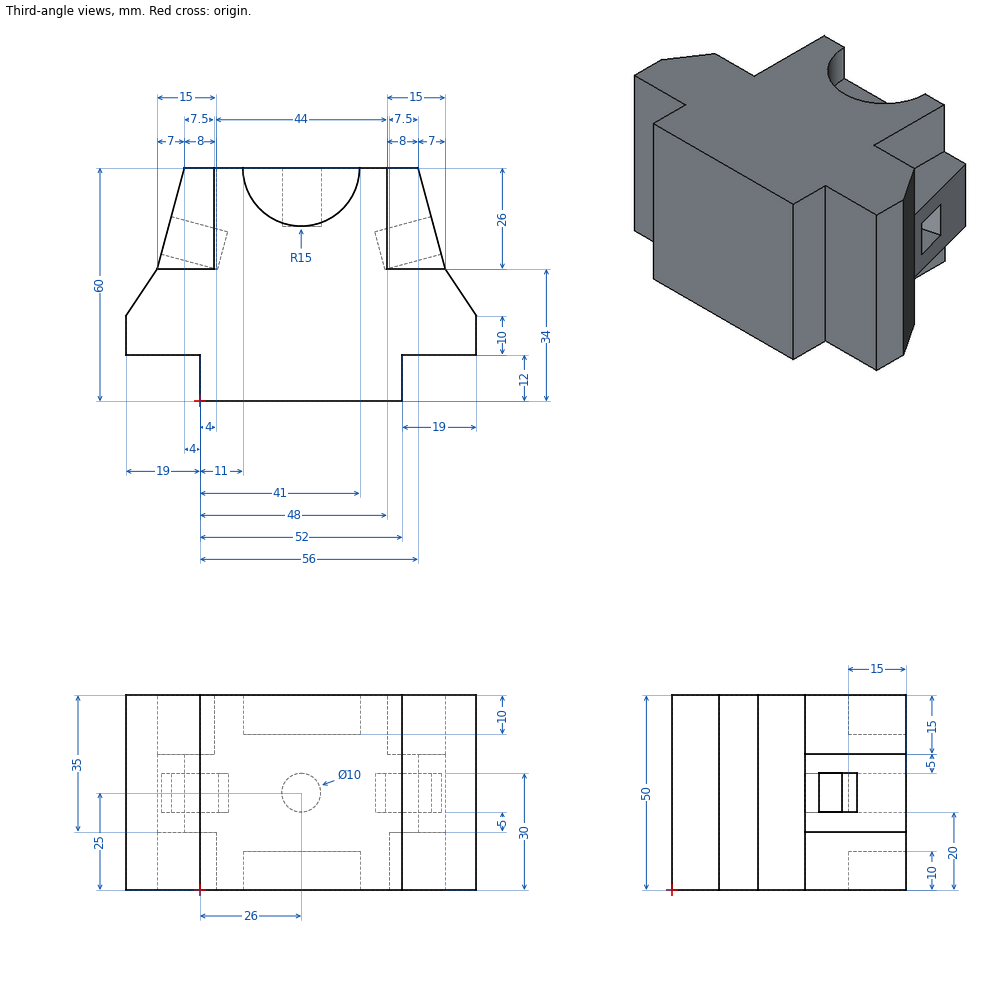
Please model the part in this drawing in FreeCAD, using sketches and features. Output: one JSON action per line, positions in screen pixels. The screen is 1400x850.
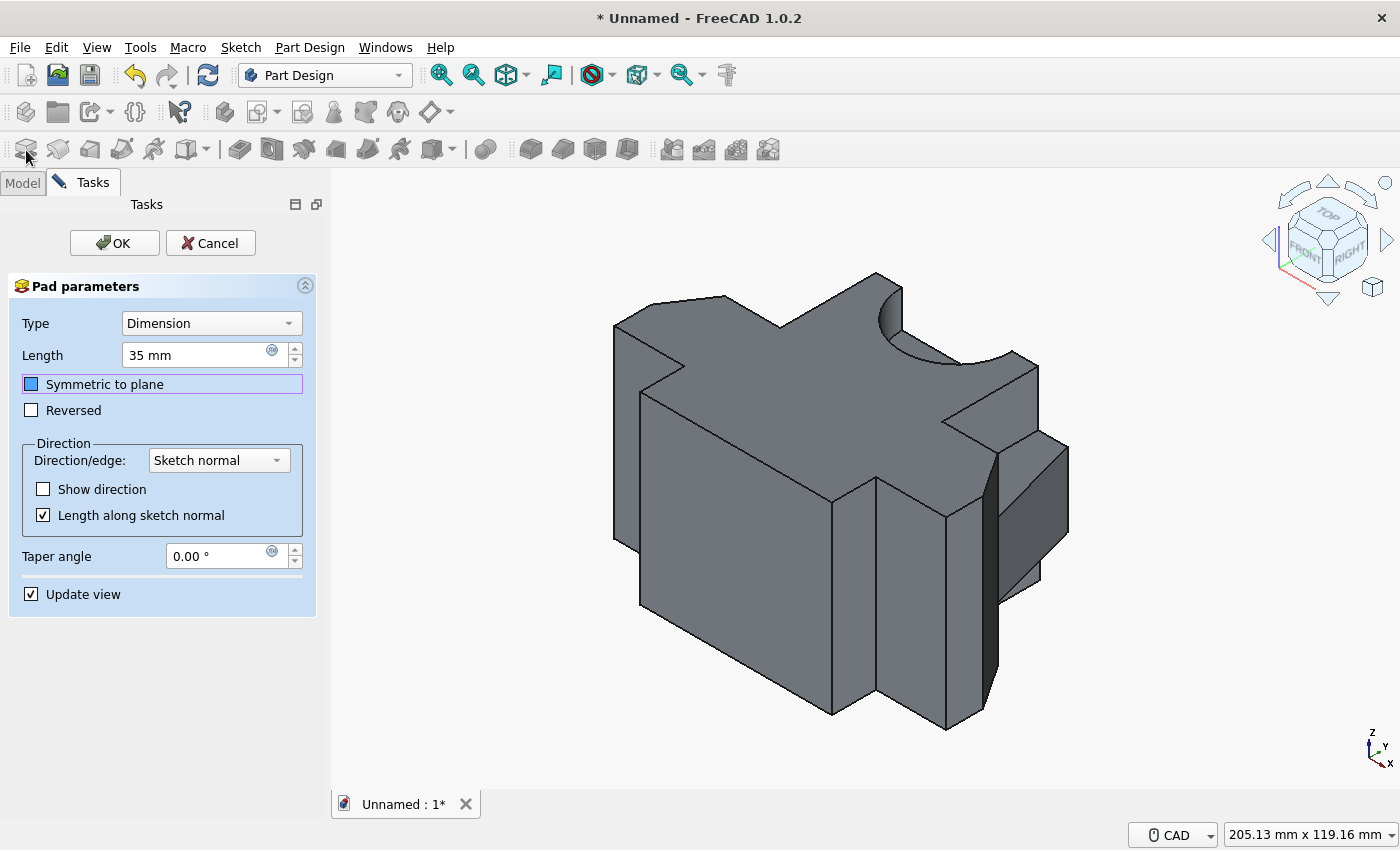
{"action": "left_click", "coordinate": [30, 410]}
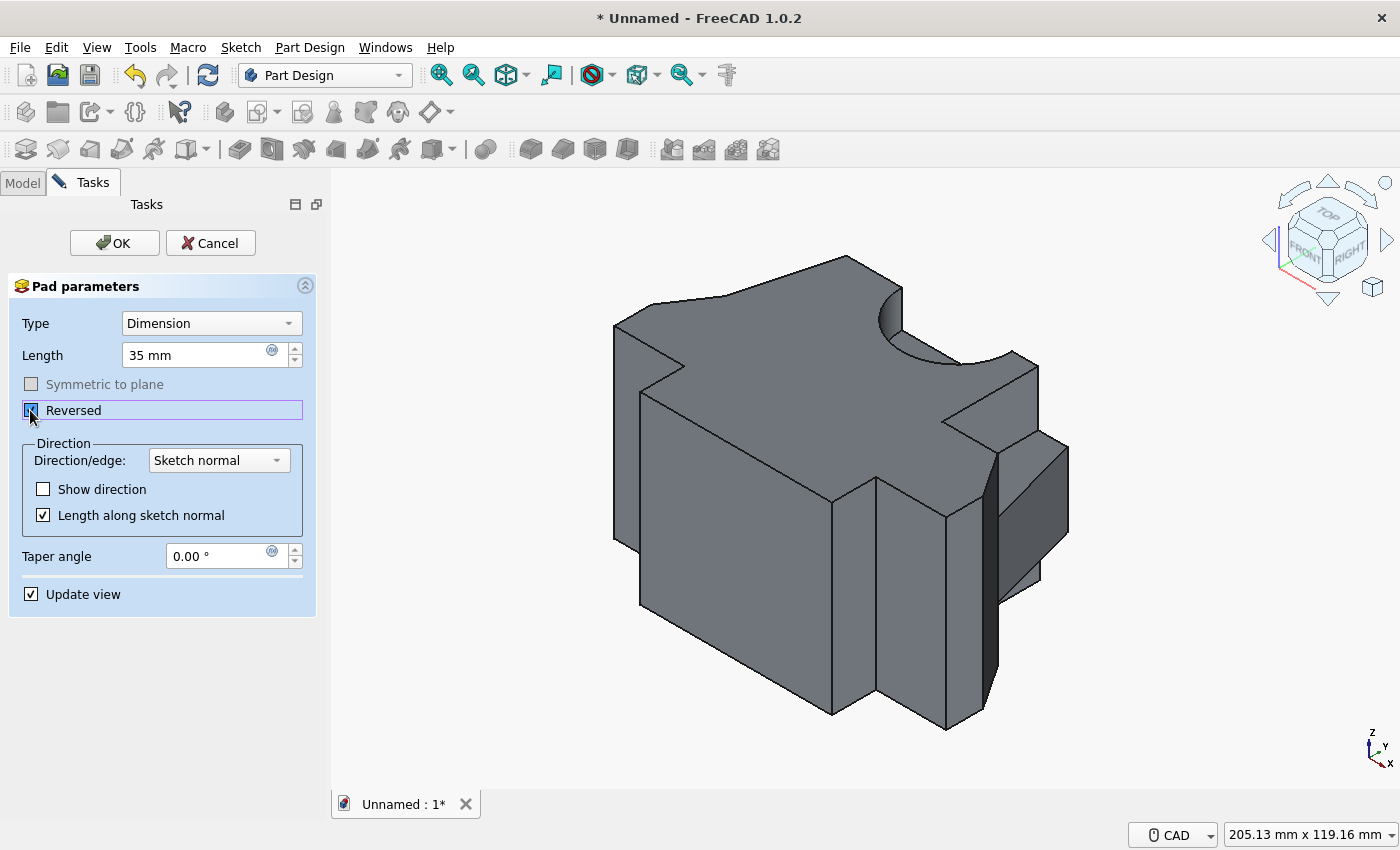
{"action": "left_click", "coordinate": [115, 243]}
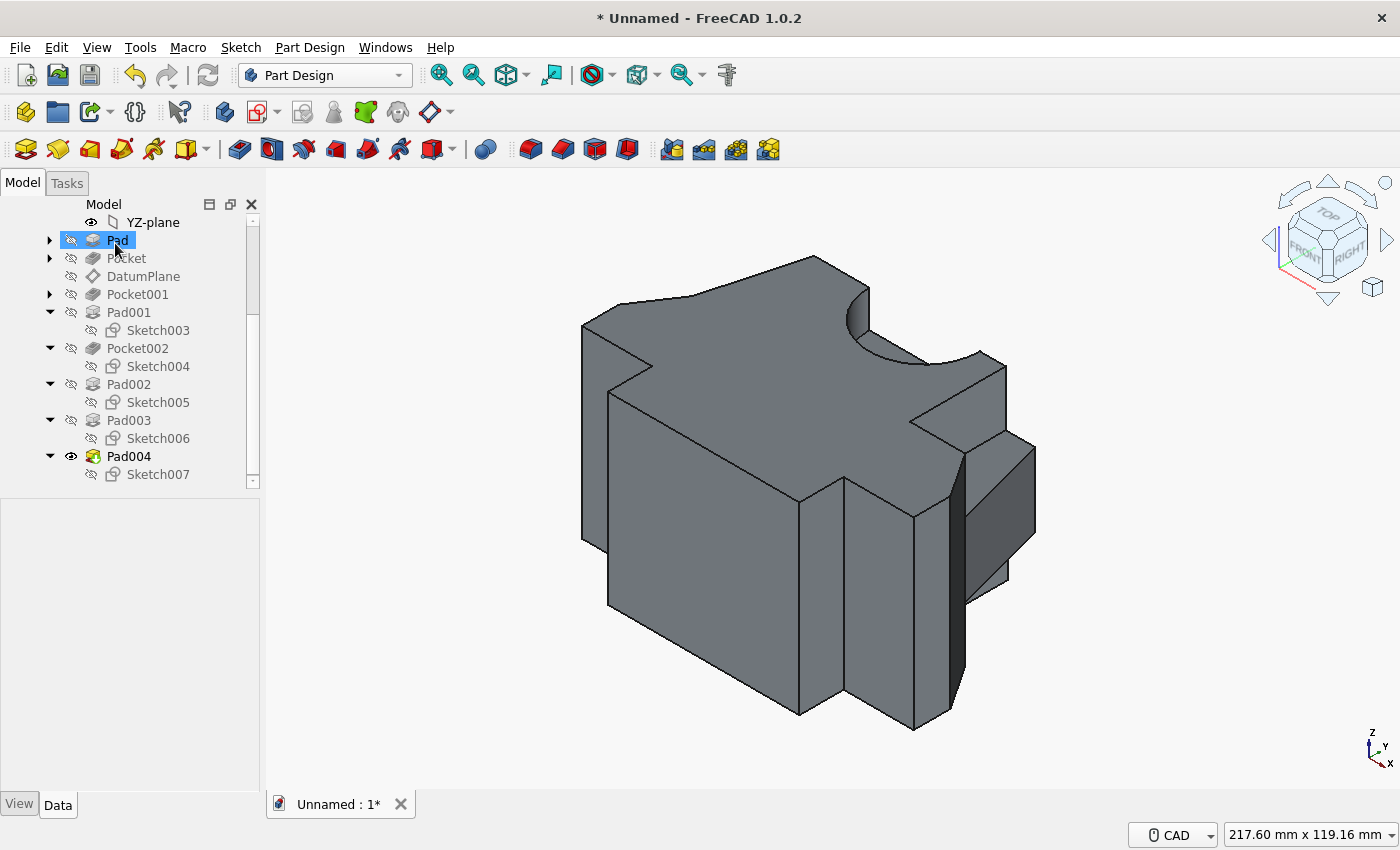
{"action": "left_click", "coordinate": [783, 401]}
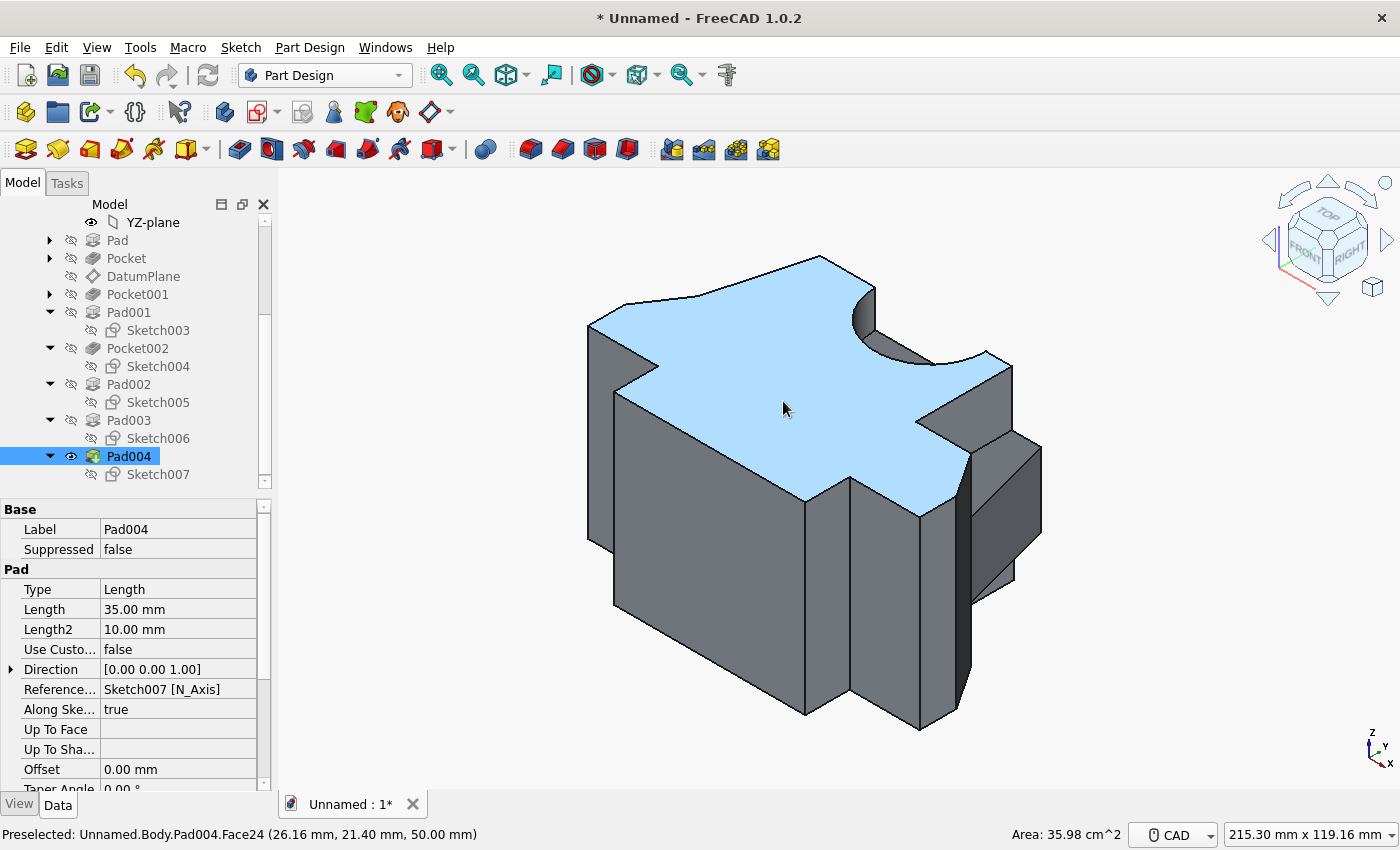
{"action": "left_click", "coordinate": [258, 112]}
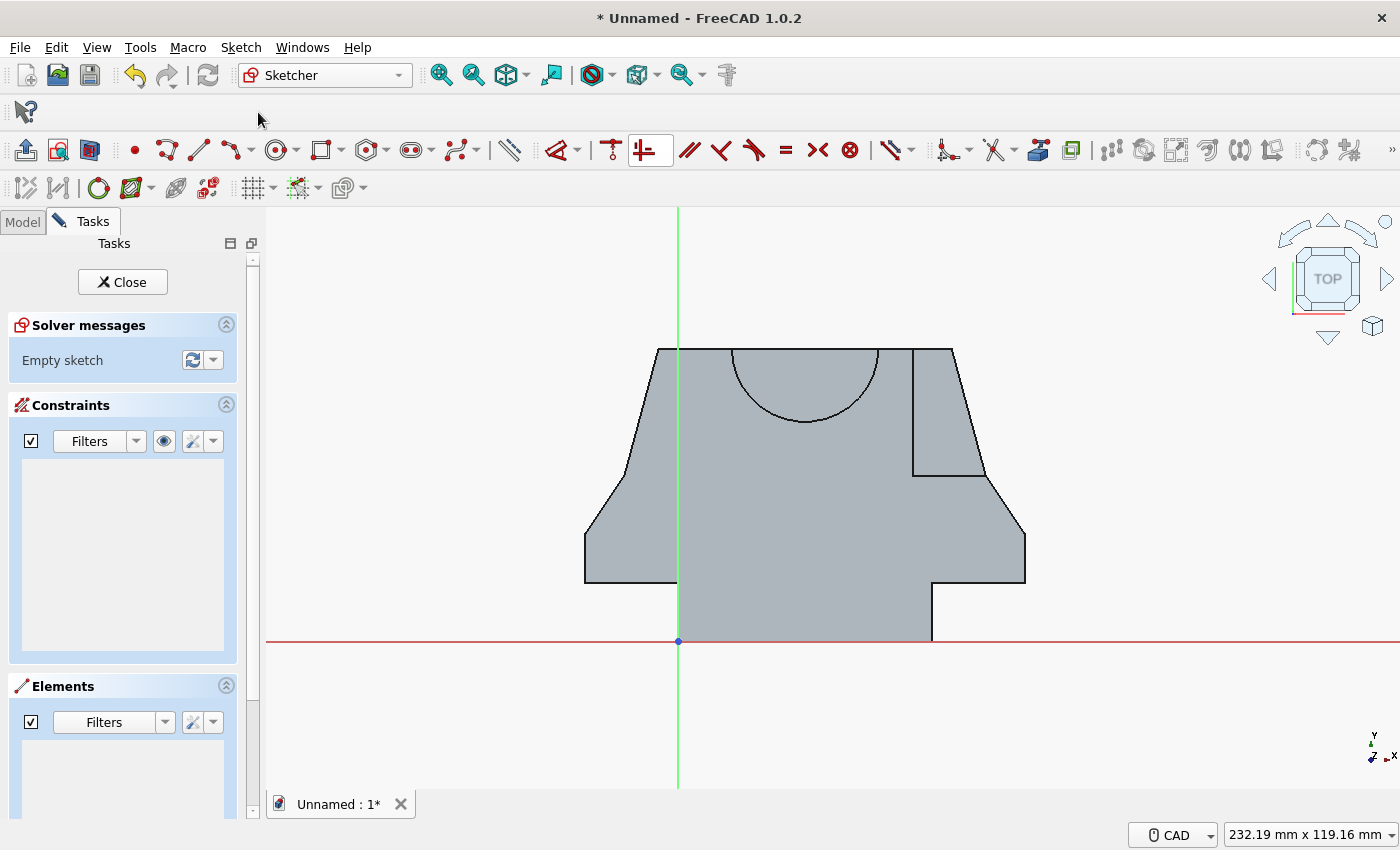
{"action": "left_click", "coordinate": [168, 150]}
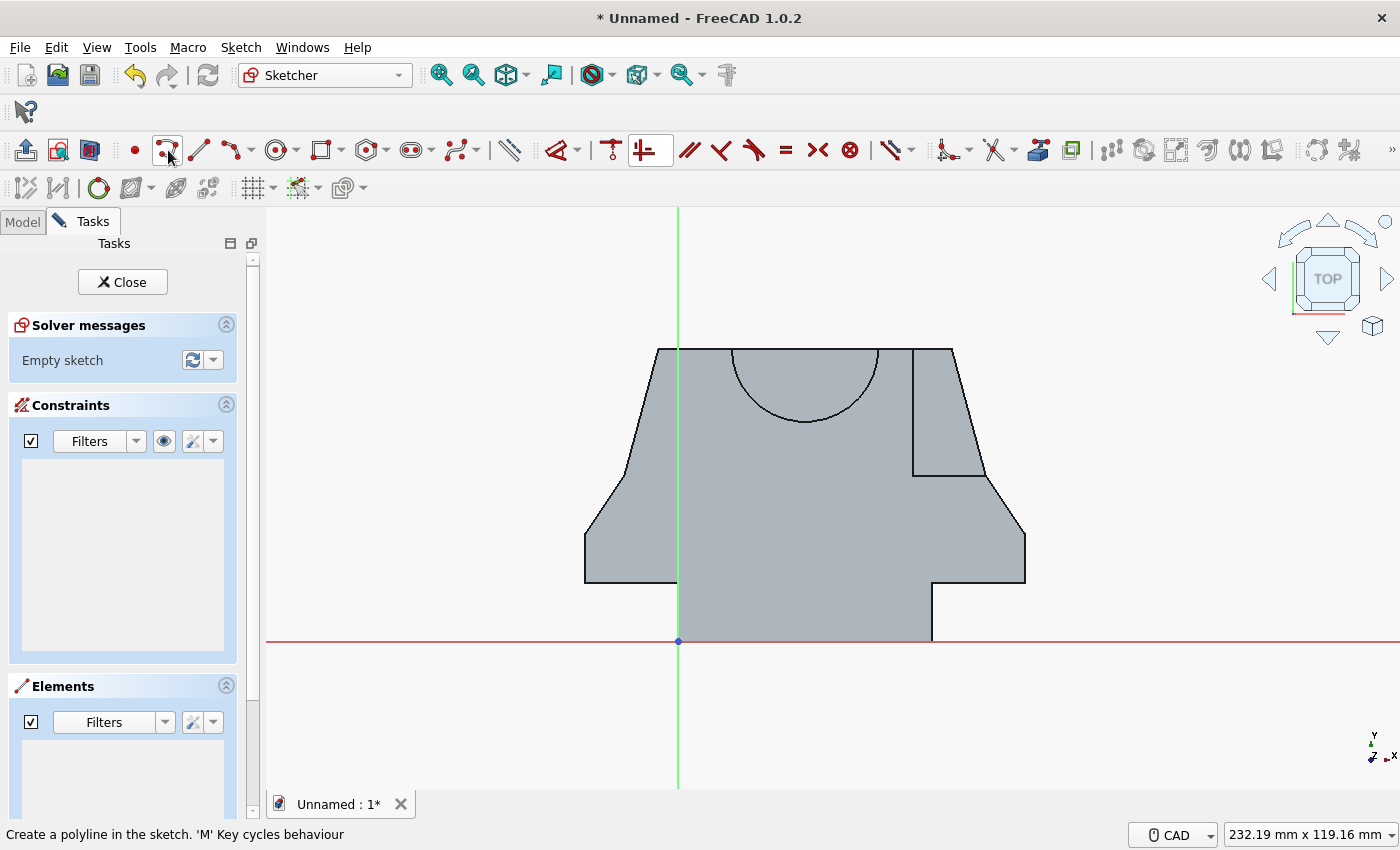
{"action": "left_click", "coordinate": [695, 476]}
{"action": "left_click", "coordinate": [695, 349]}
{"action": "left_click", "coordinate": [659, 349]}
{"action": "left_click", "coordinate": [624, 476]}
{"action": "left_click", "coordinate": [695, 477]}
{"action": "key", "text": "Escape"}
{"action": "key", "text": "Escape"}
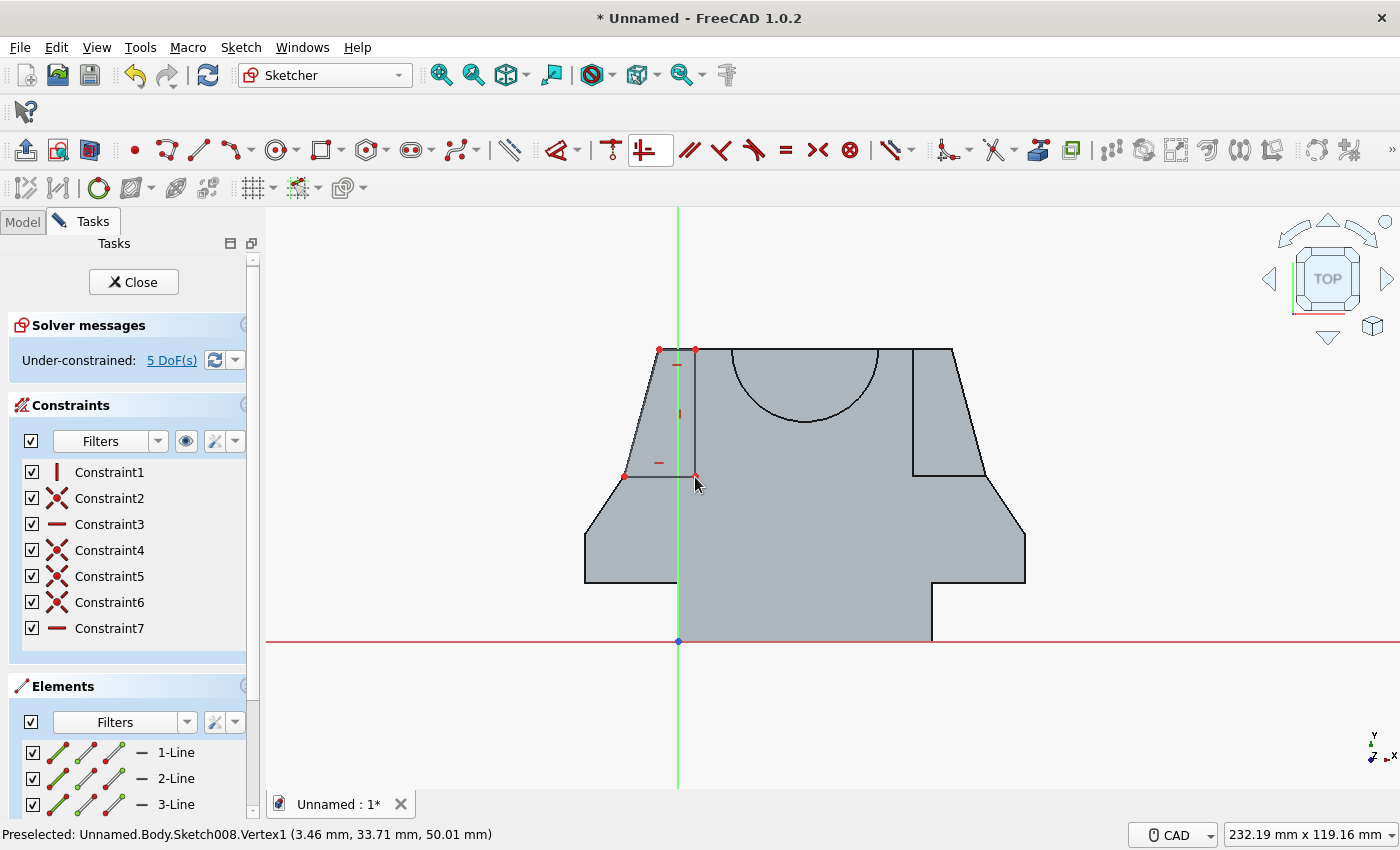
{"action": "left_click", "coordinate": [556, 150]}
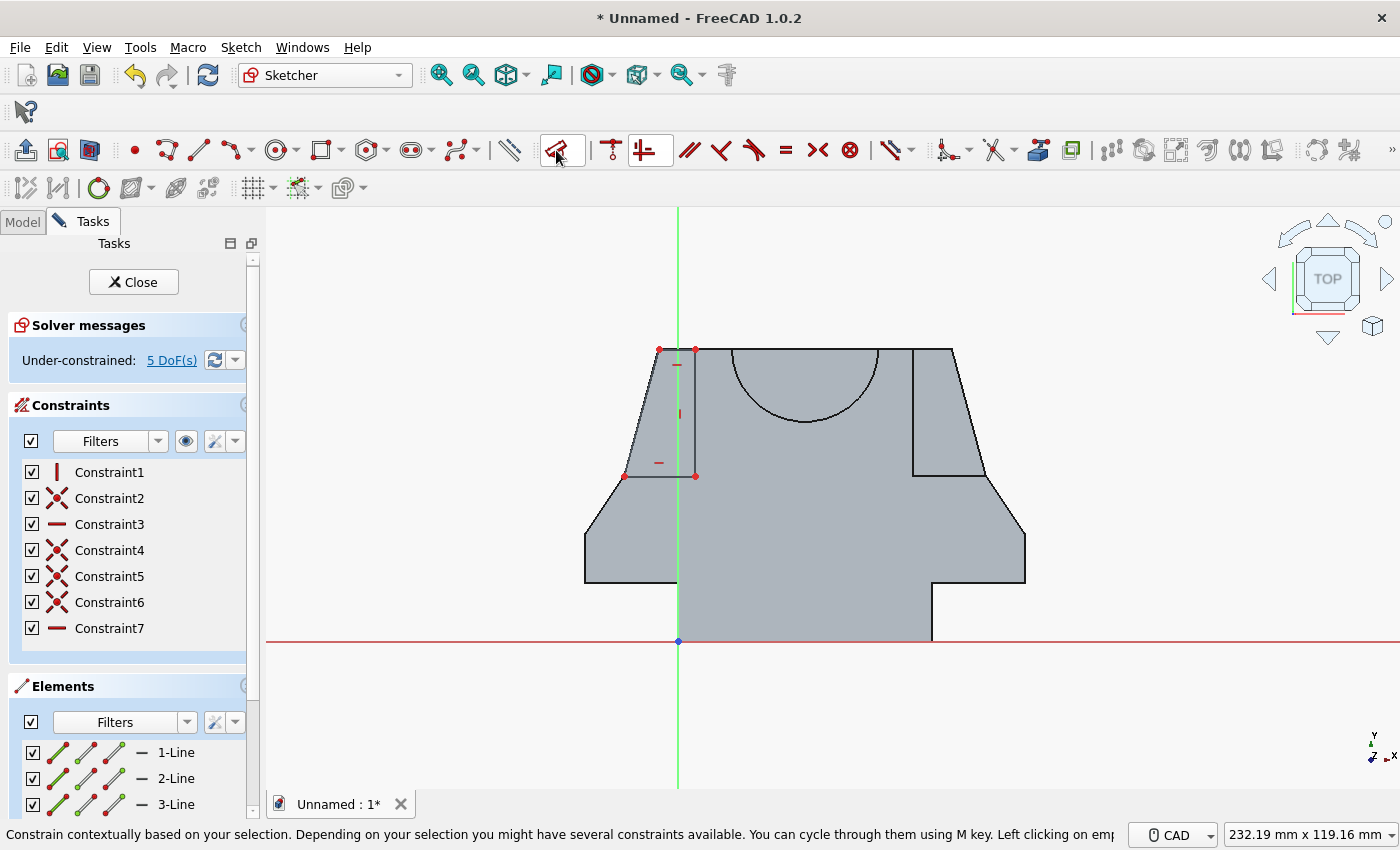
{"action": "left_click", "coordinate": [695, 439]}
{"action": "left_click", "coordinate": [729, 414]}